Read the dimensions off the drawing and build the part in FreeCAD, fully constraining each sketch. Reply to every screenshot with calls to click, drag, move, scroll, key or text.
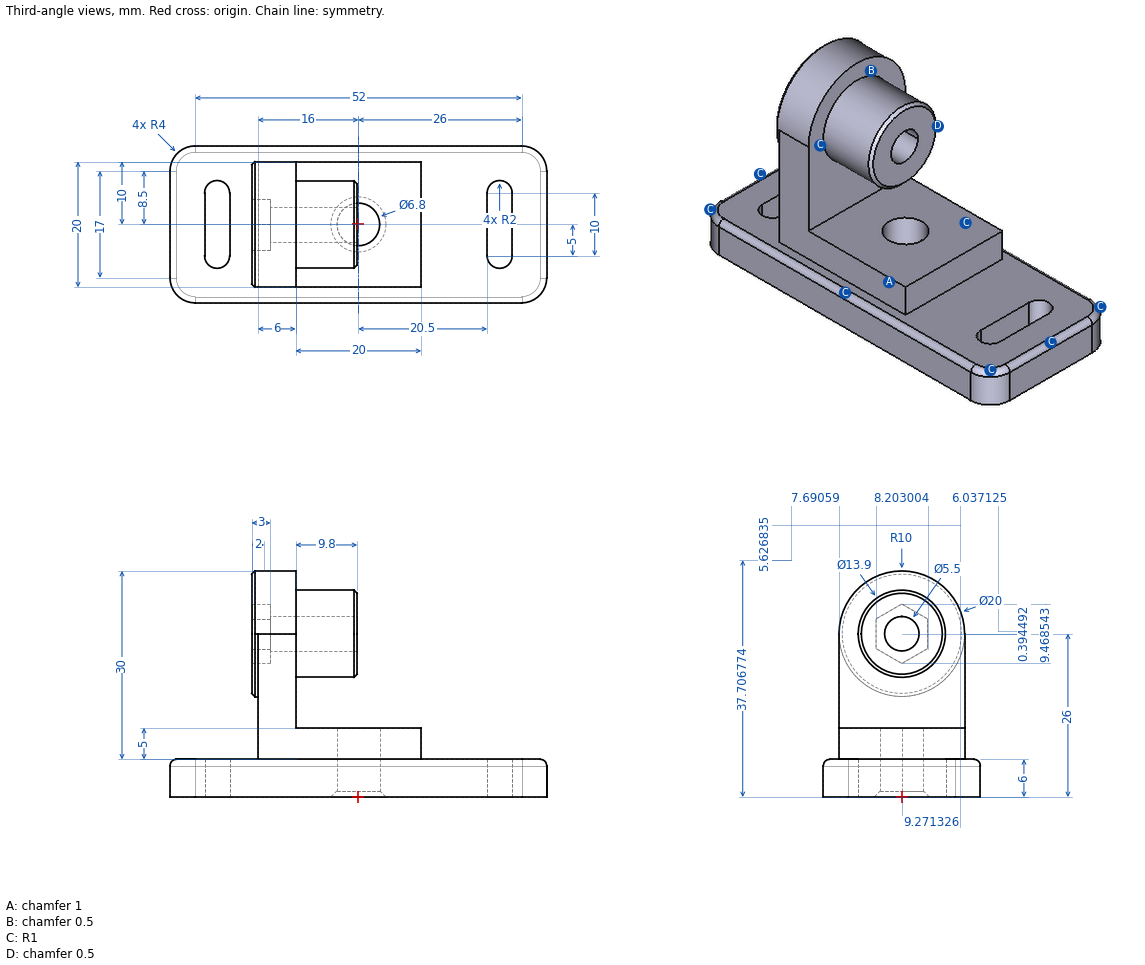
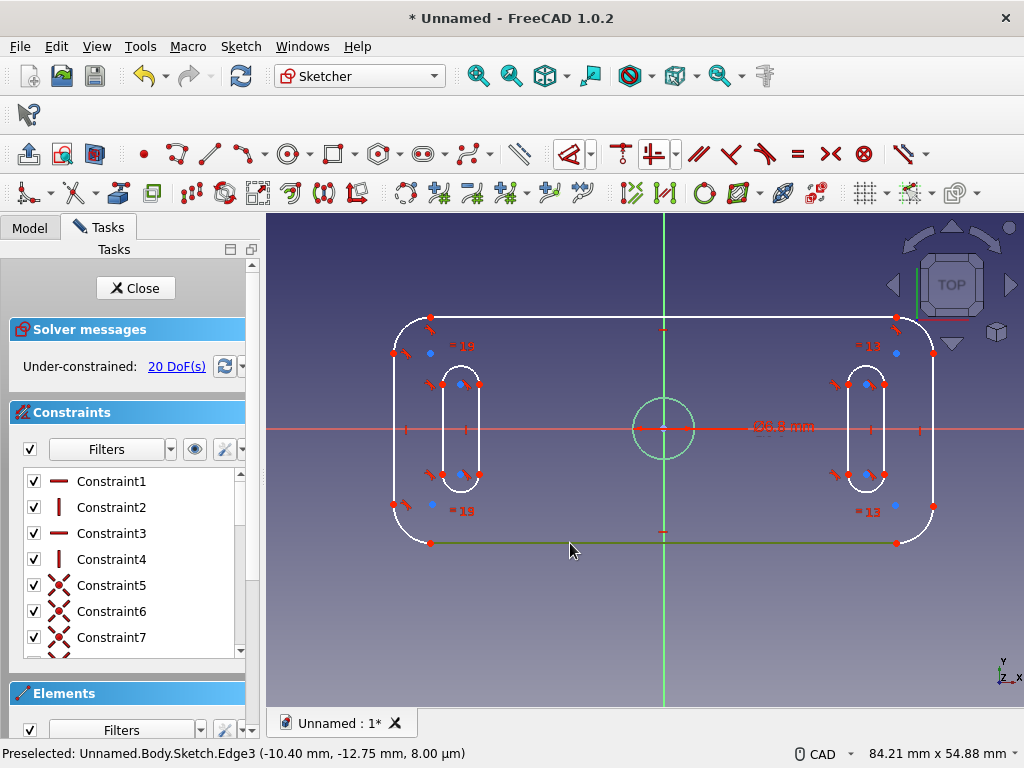
click(398, 522)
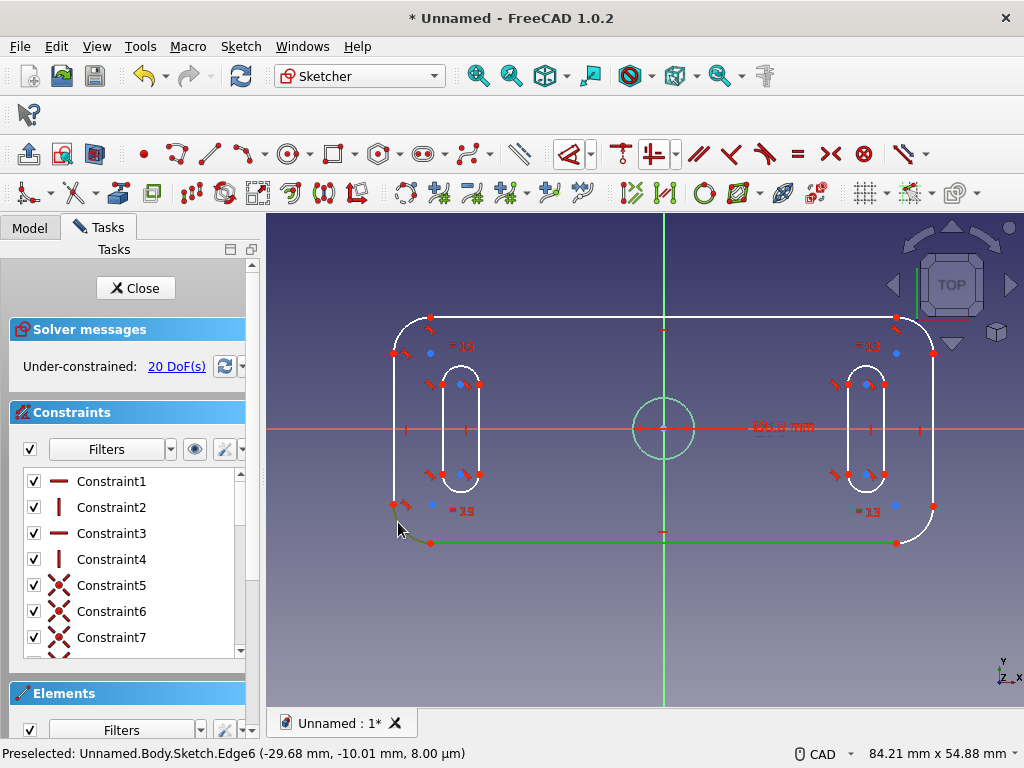
click(765, 154)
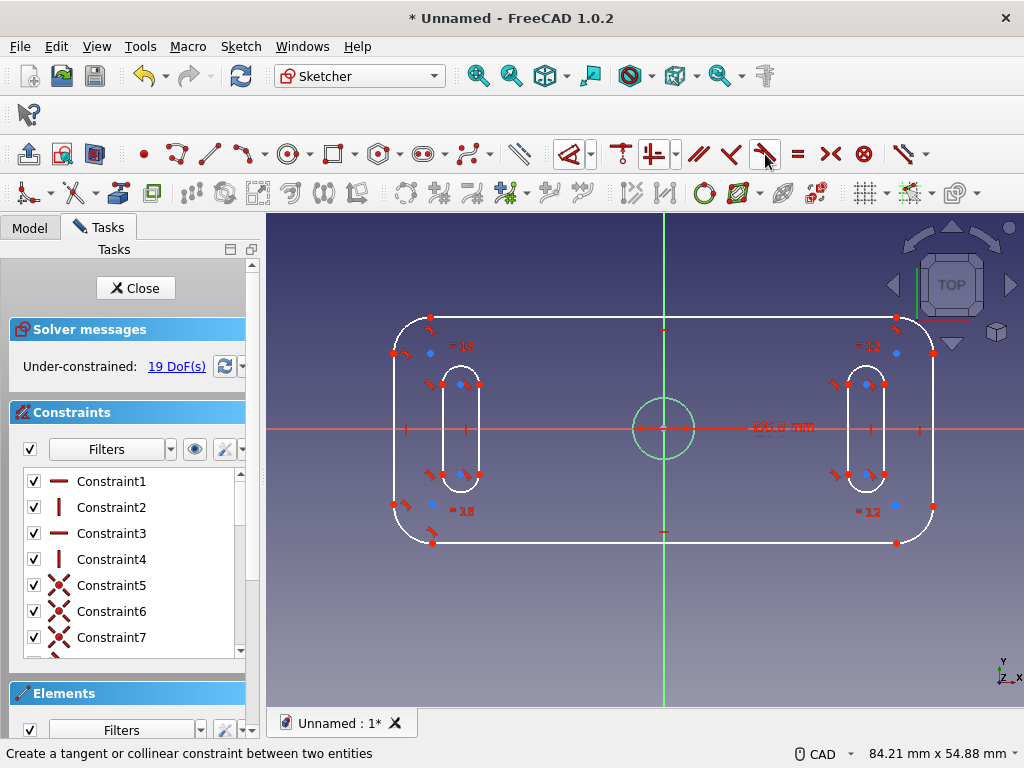
click(572, 543)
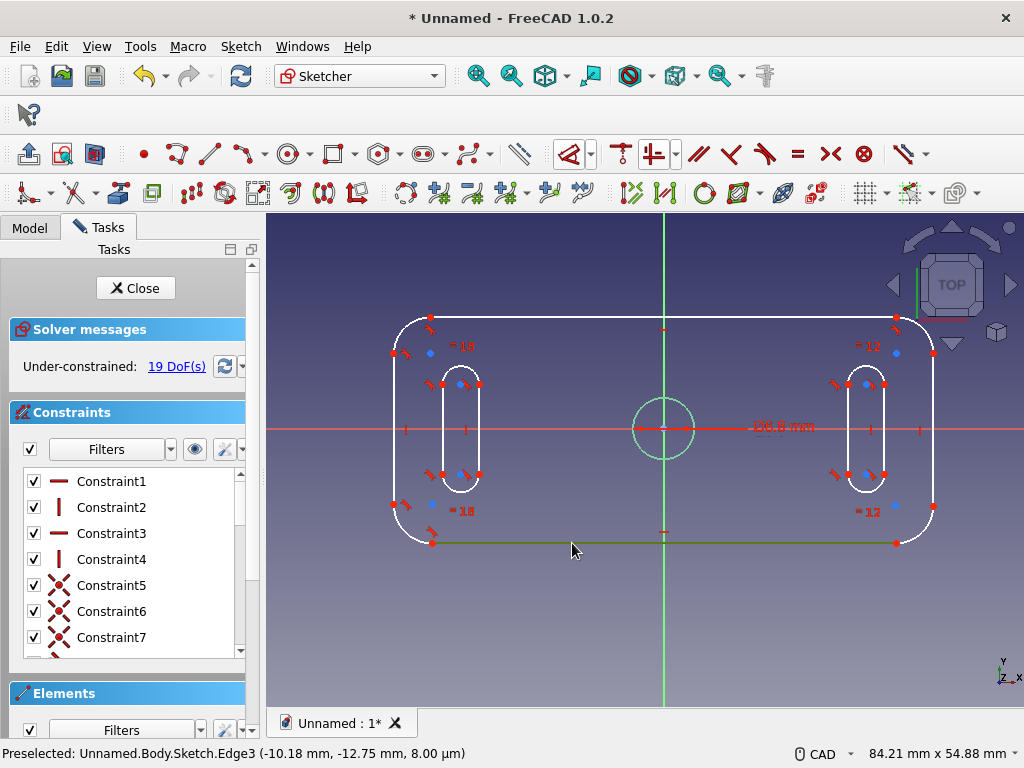
scroll(399, 524, down, 2)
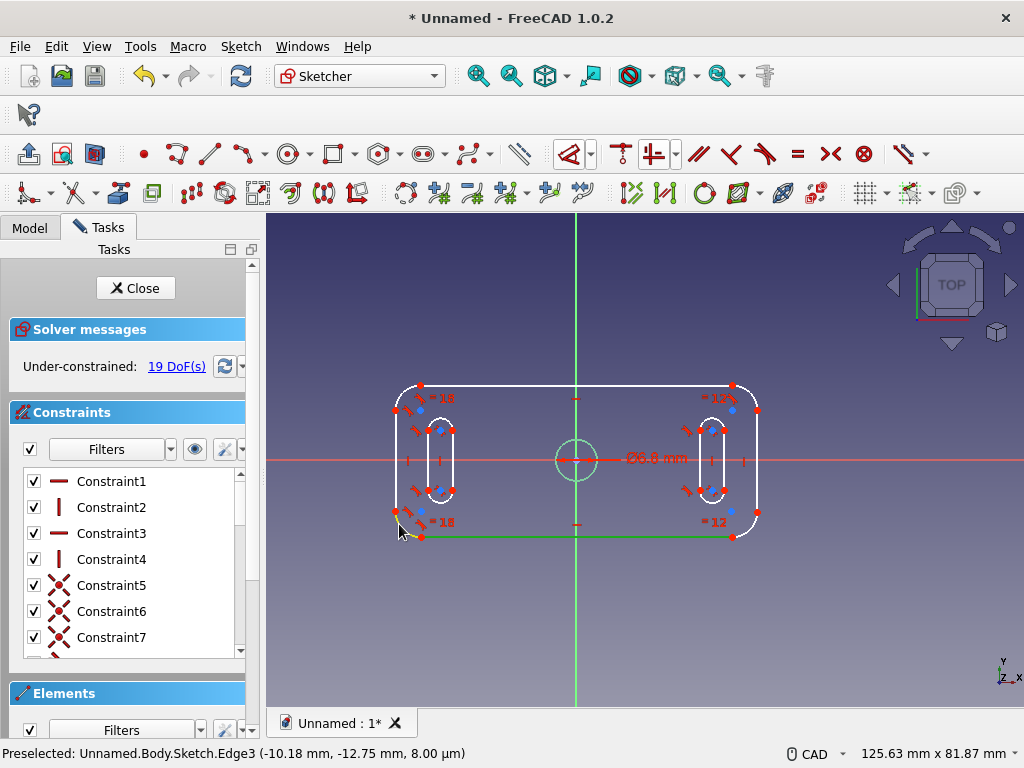
scroll(744, 534, up, 2)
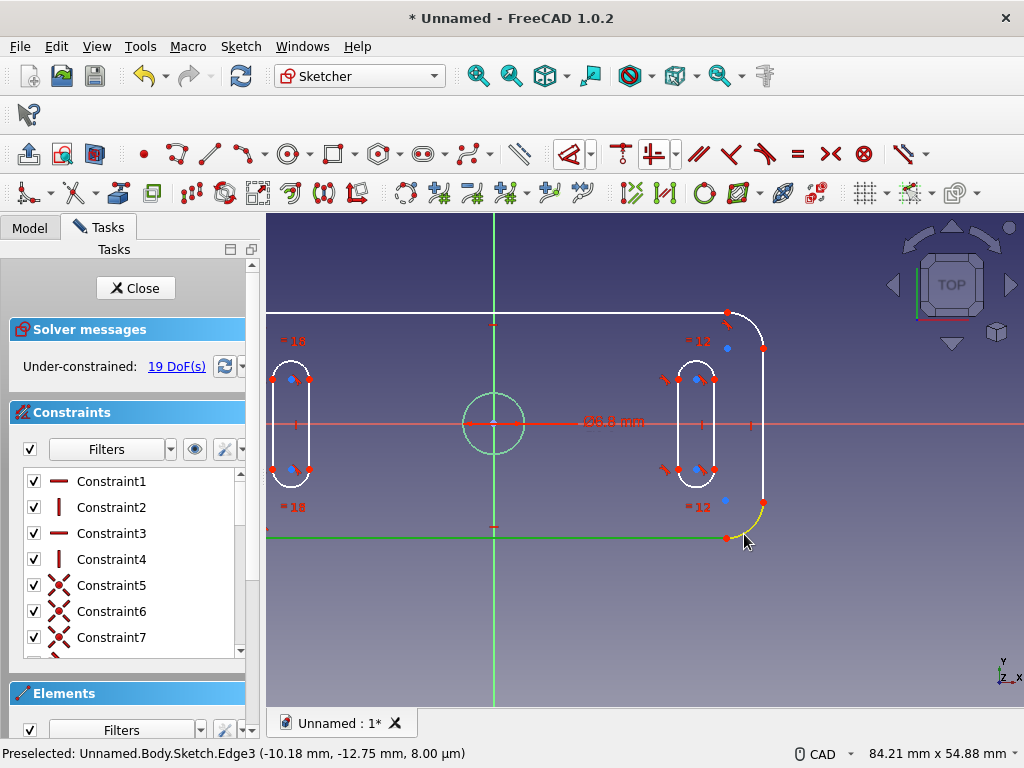
click(743, 534)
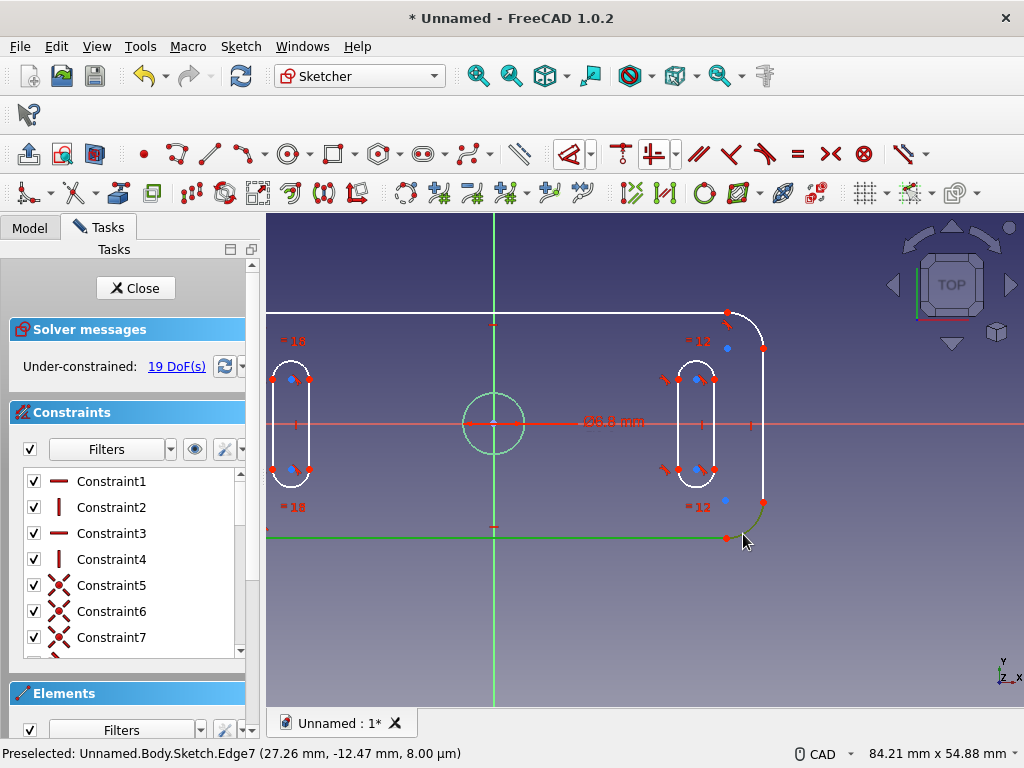
click(765, 154)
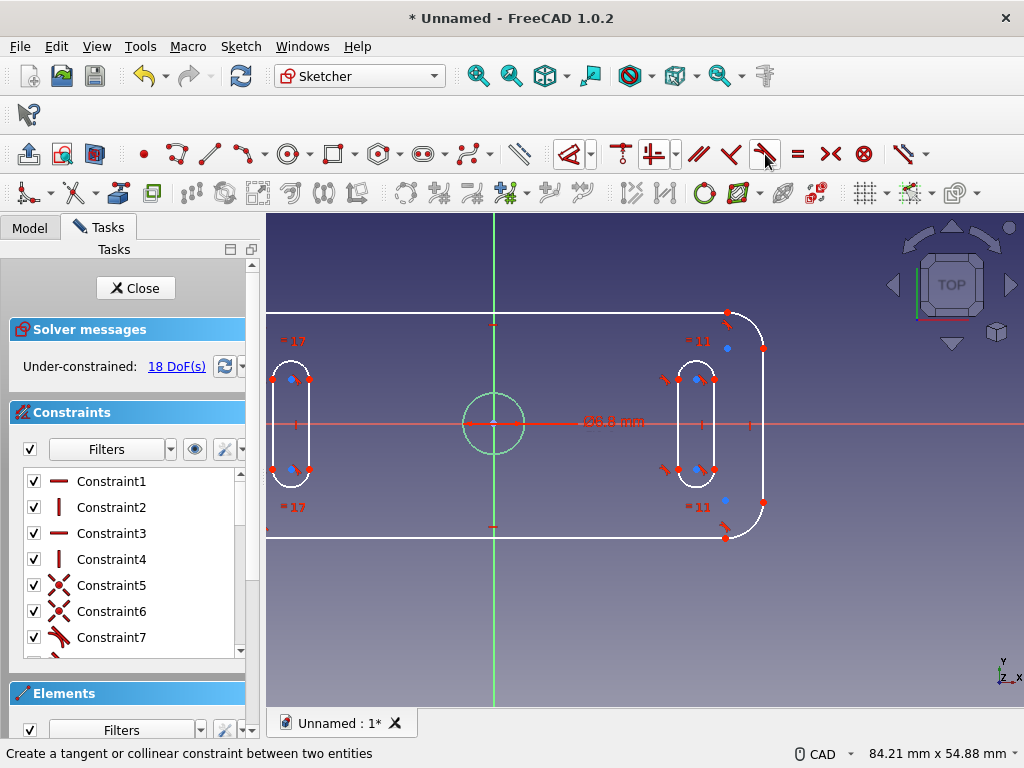
click(763, 456)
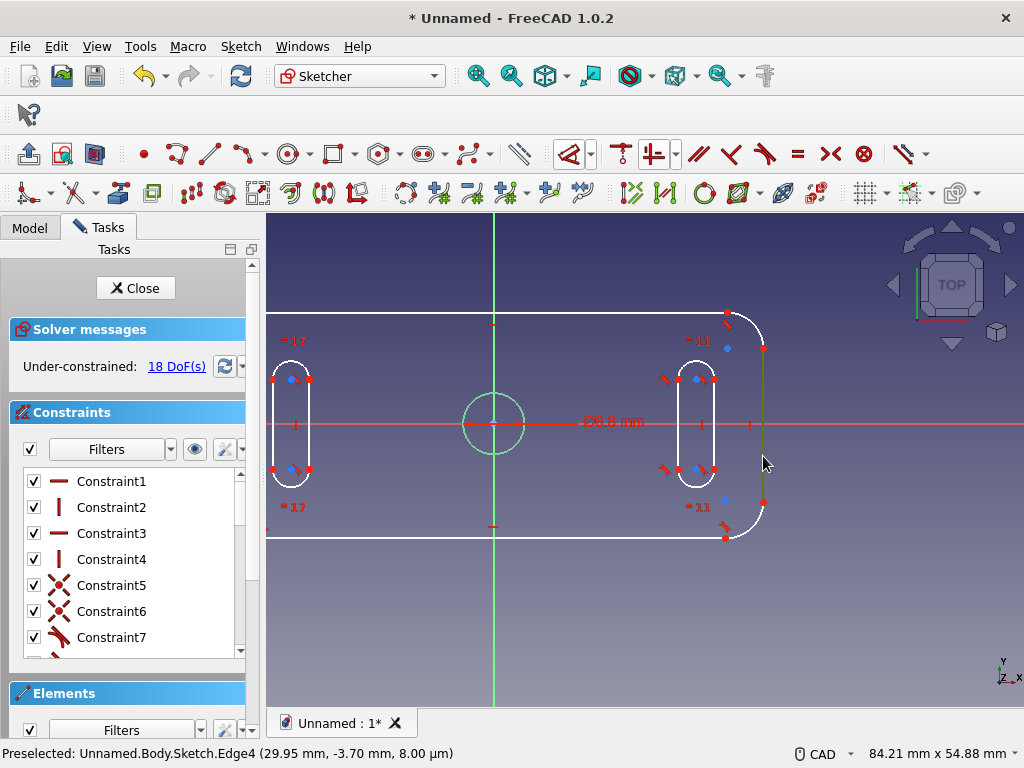
click(742, 535)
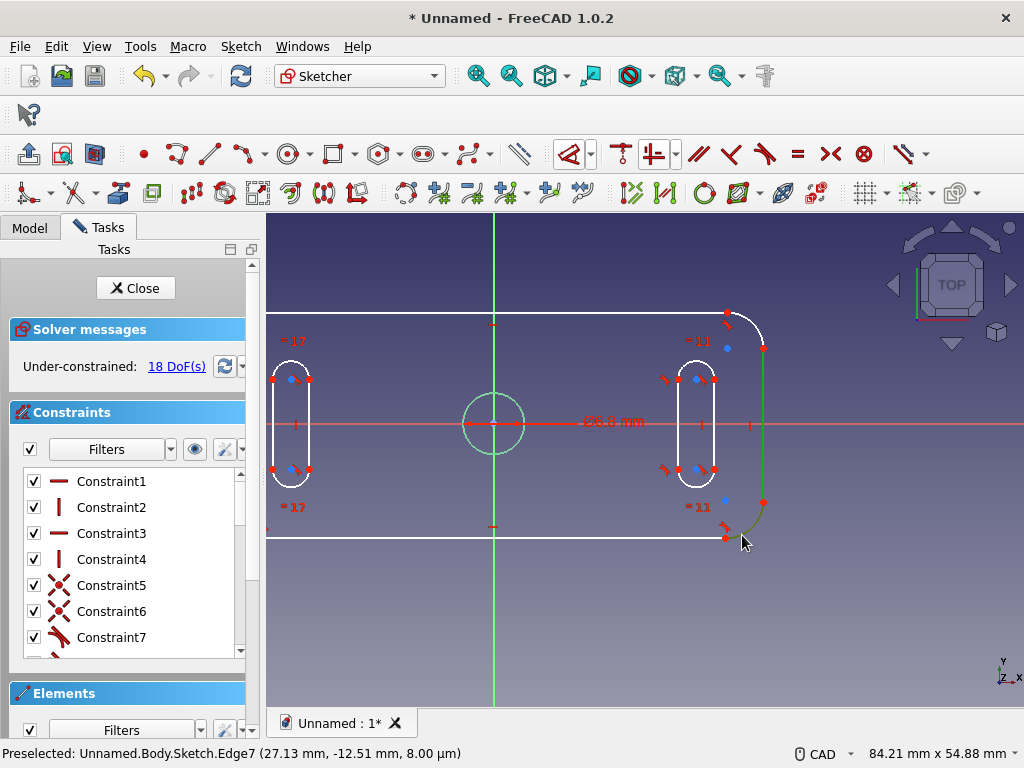
click(765, 154)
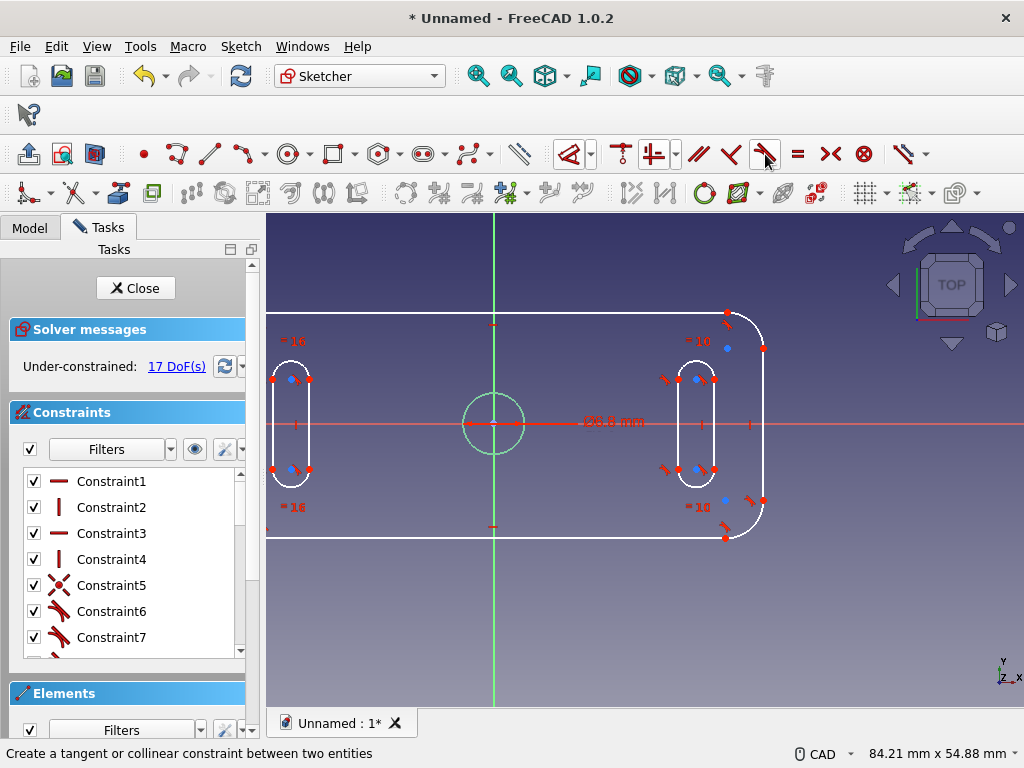
click(763, 455)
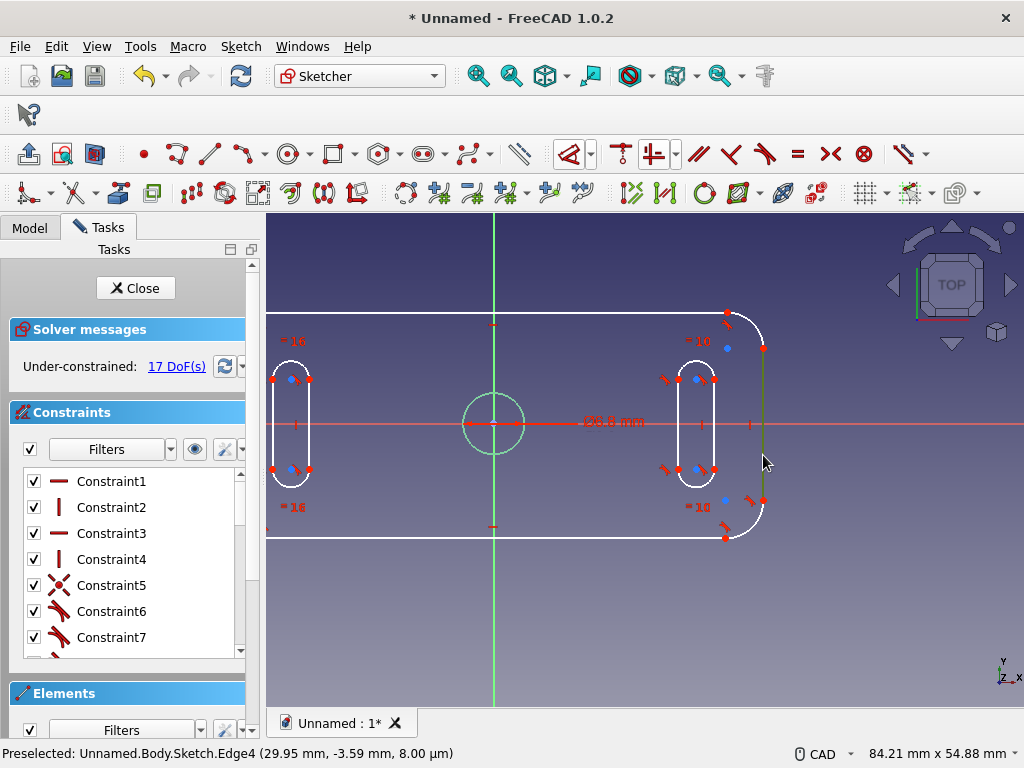
click(759, 332)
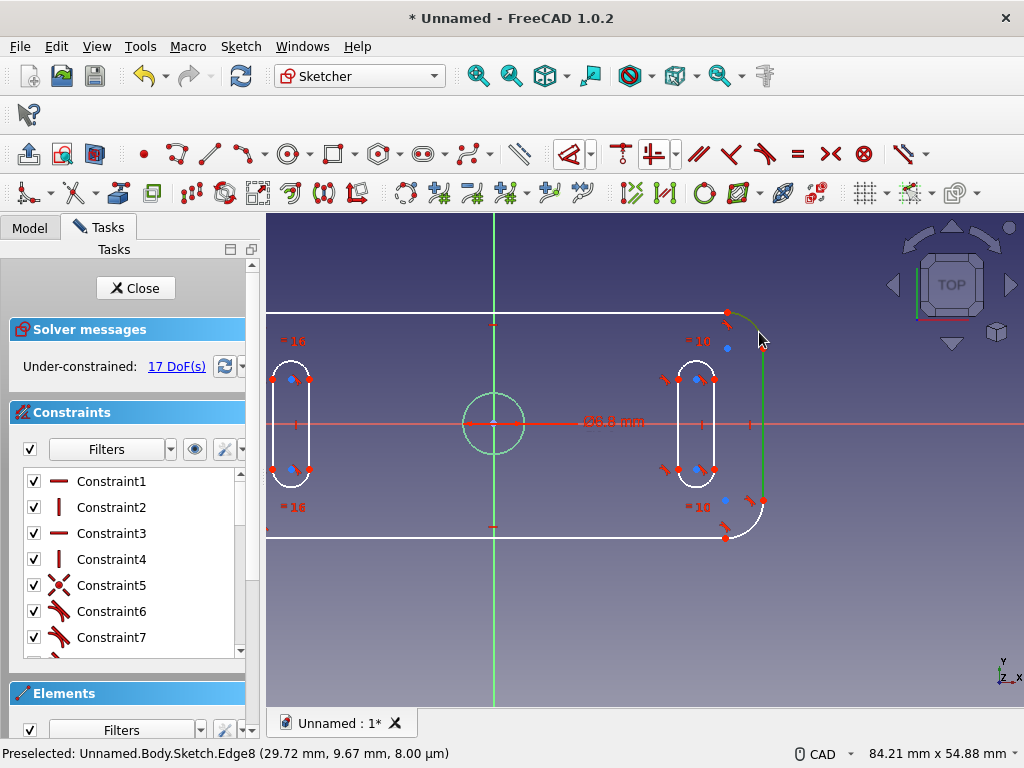
click(765, 154)